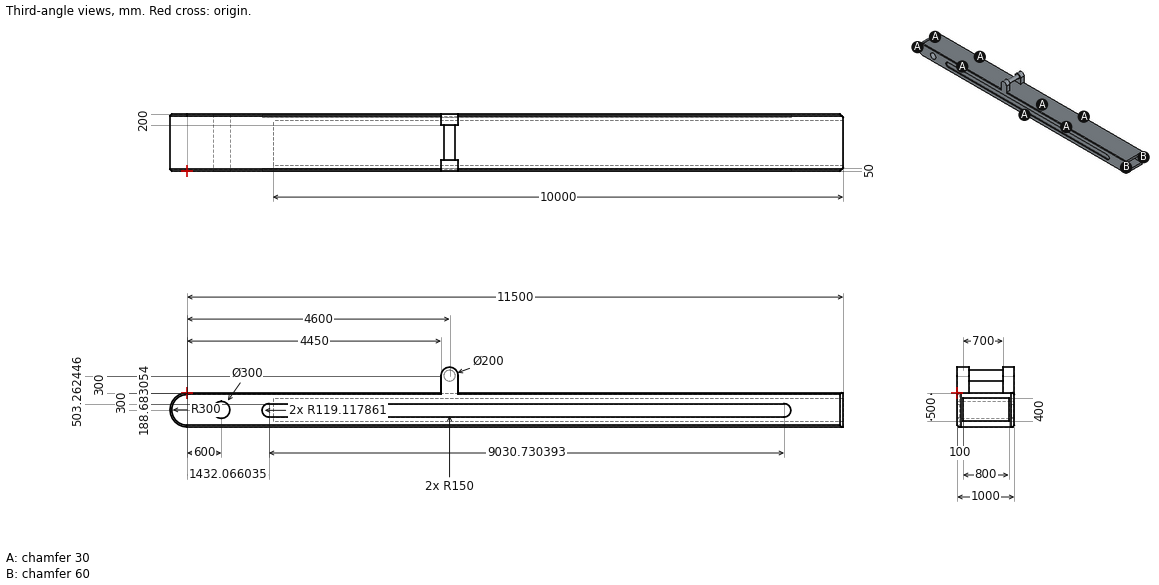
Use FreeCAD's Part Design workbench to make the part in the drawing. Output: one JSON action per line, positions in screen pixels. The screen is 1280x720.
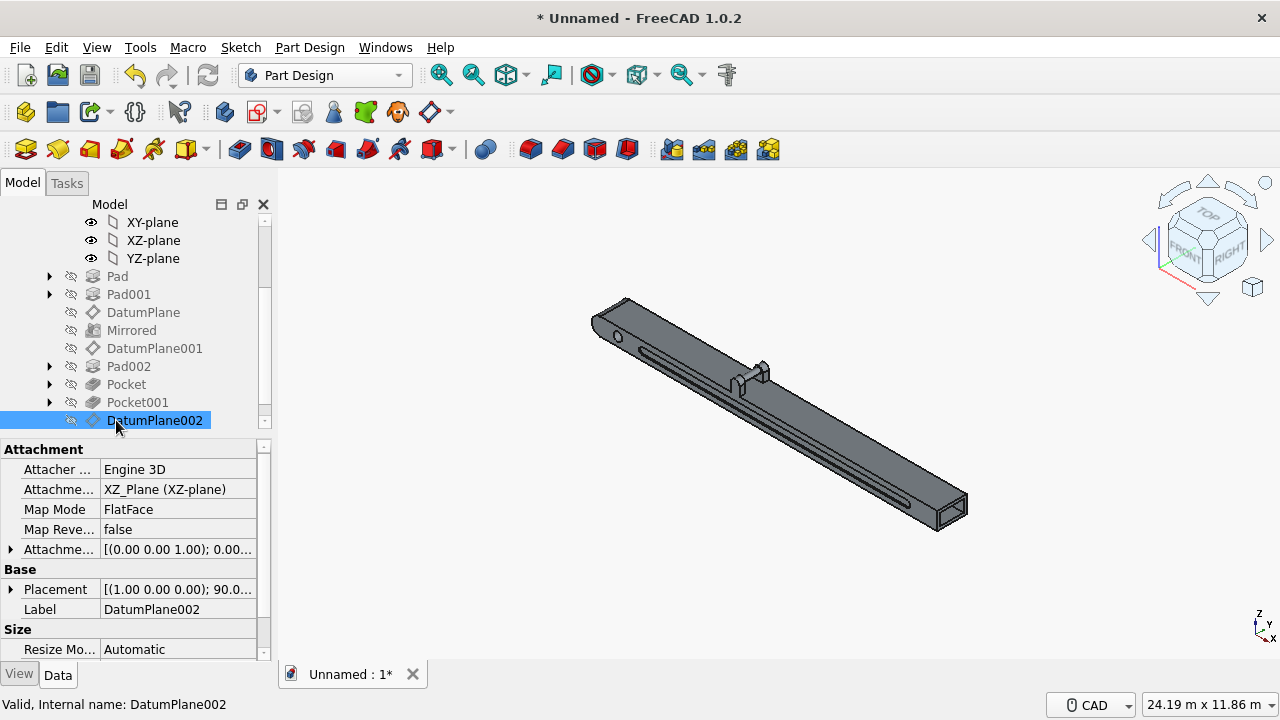
{"action": "left_click", "coordinate": [838, 453]}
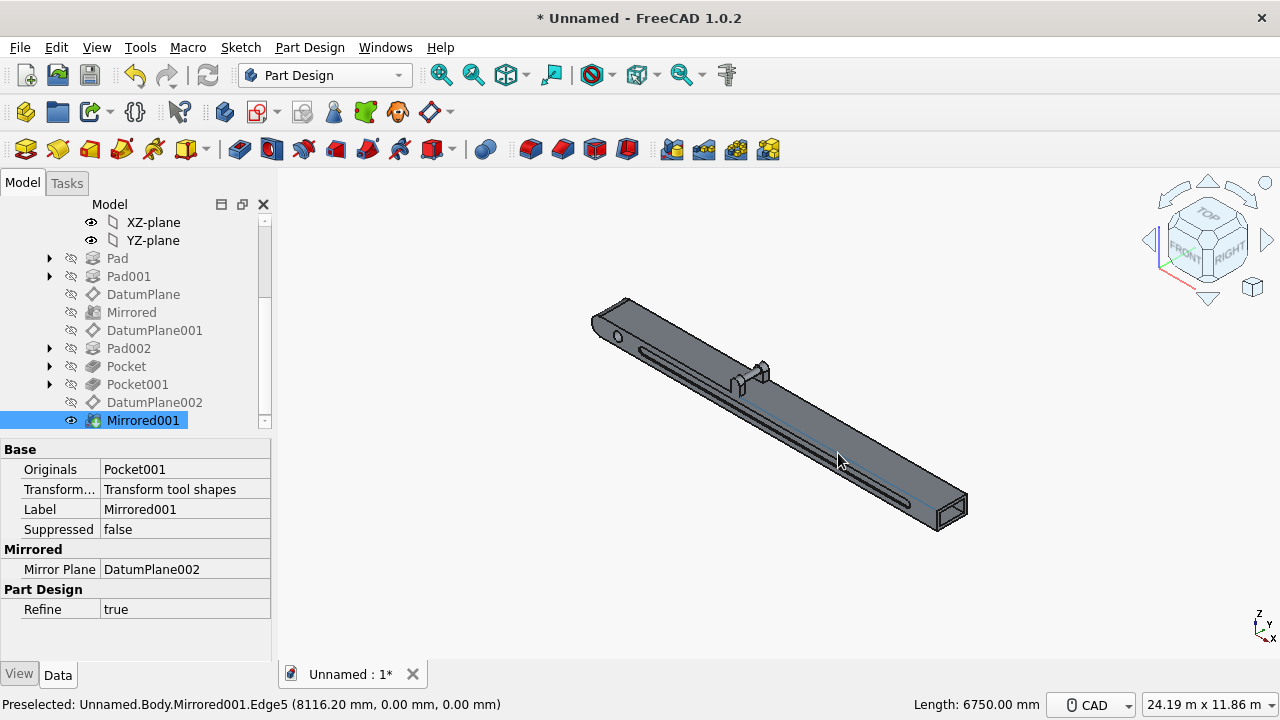
{"action": "left_click", "coordinate": [666, 353], "text": "ctrl"}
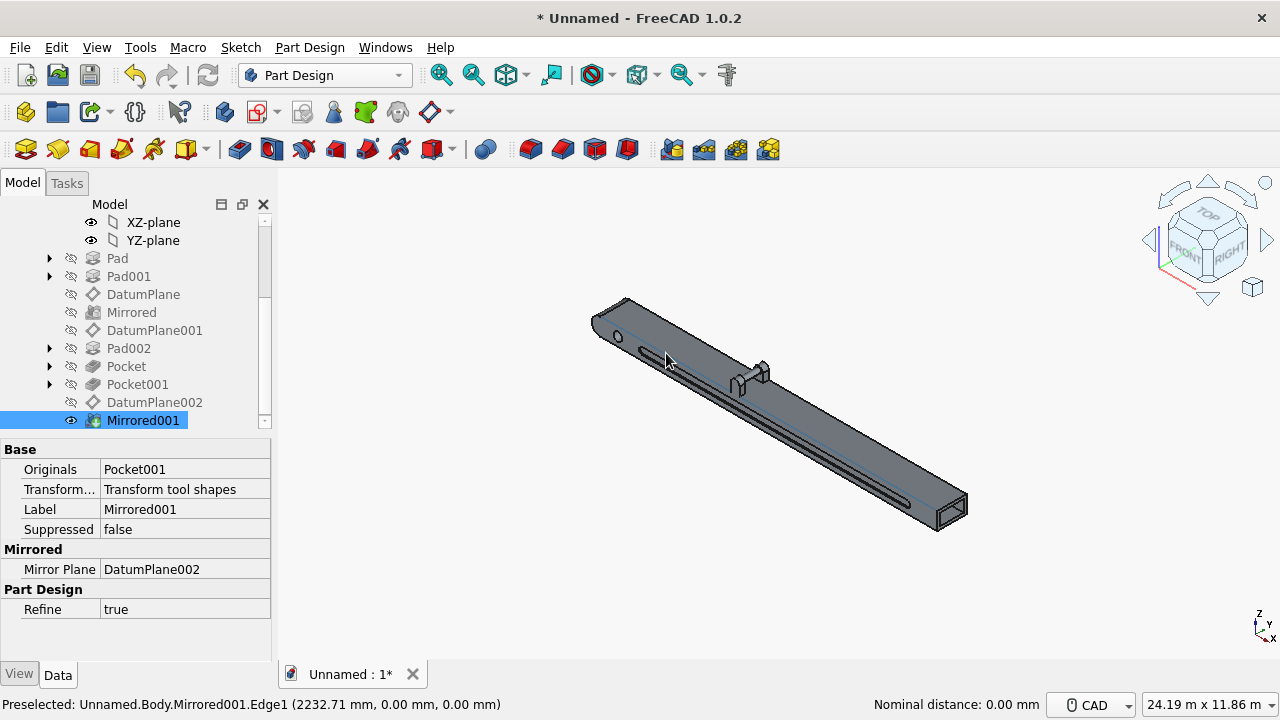
{"action": "left_click", "coordinate": [592, 321], "text": "ctrl"}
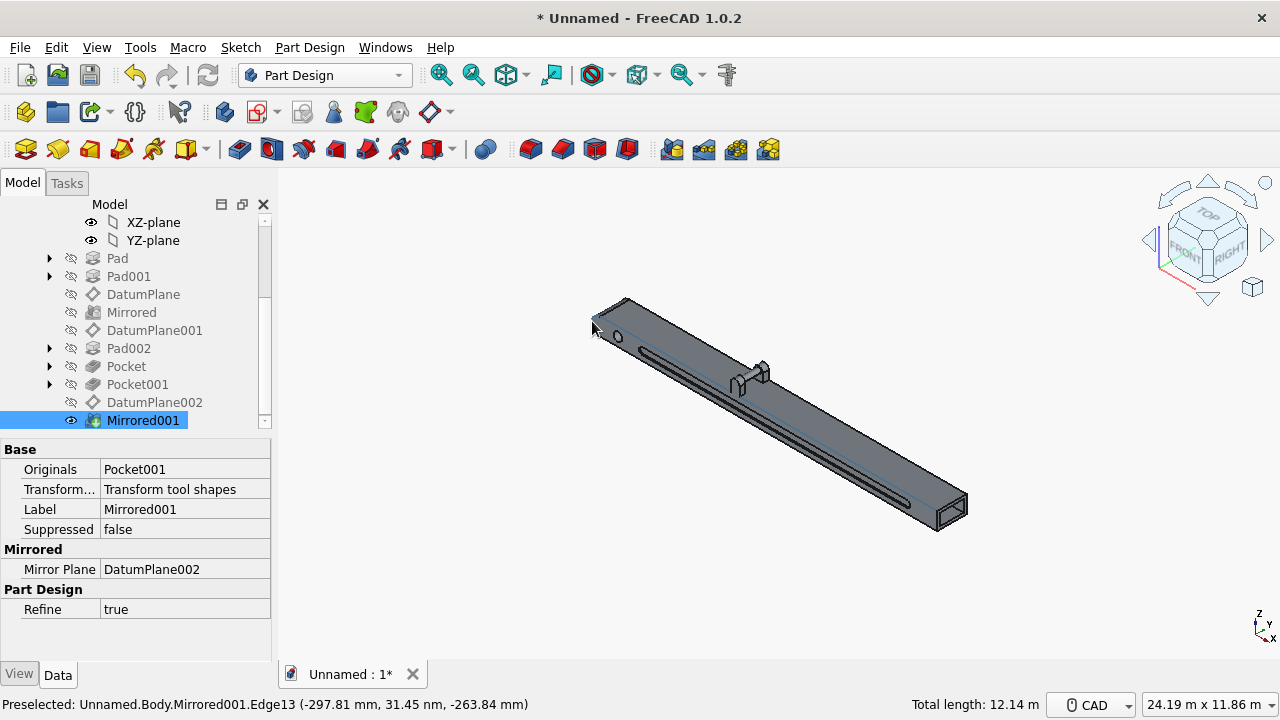
{"action": "key", "text": "2"}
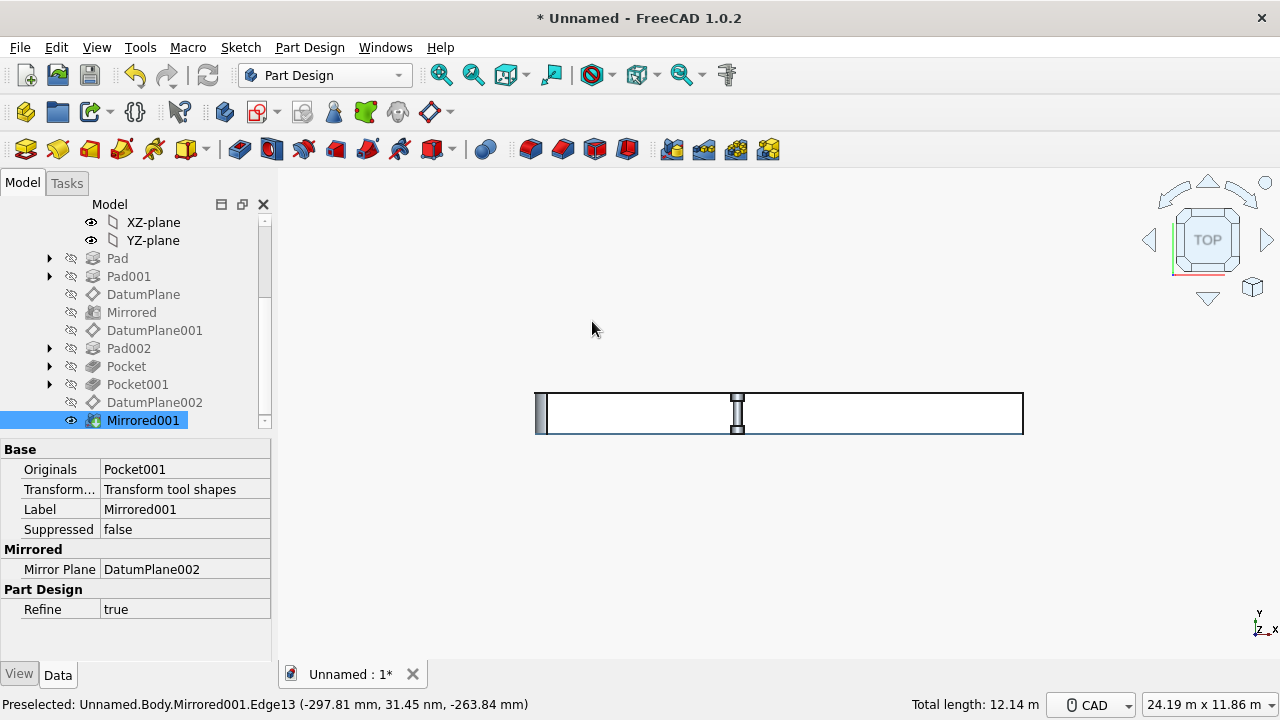
{"action": "left_click", "coordinate": [884, 392], "text": "ctrl"}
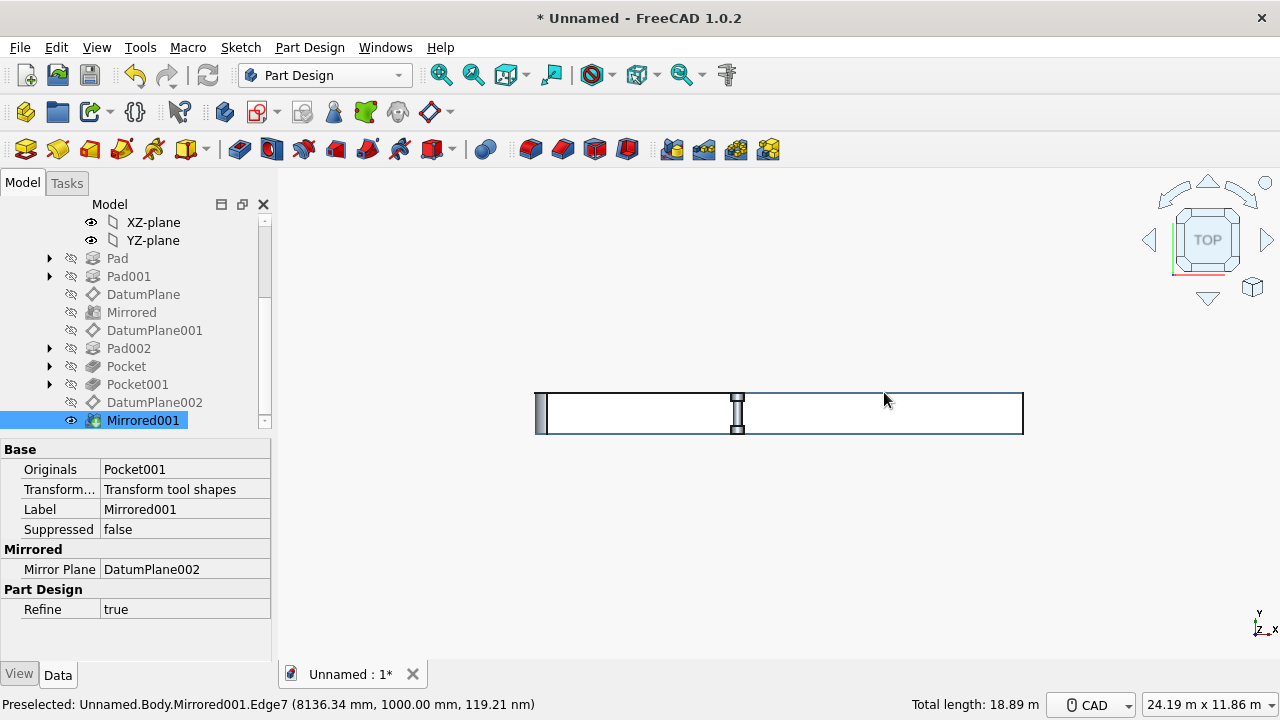
{"action": "left_click", "coordinate": [535, 392], "text": "ctrl"}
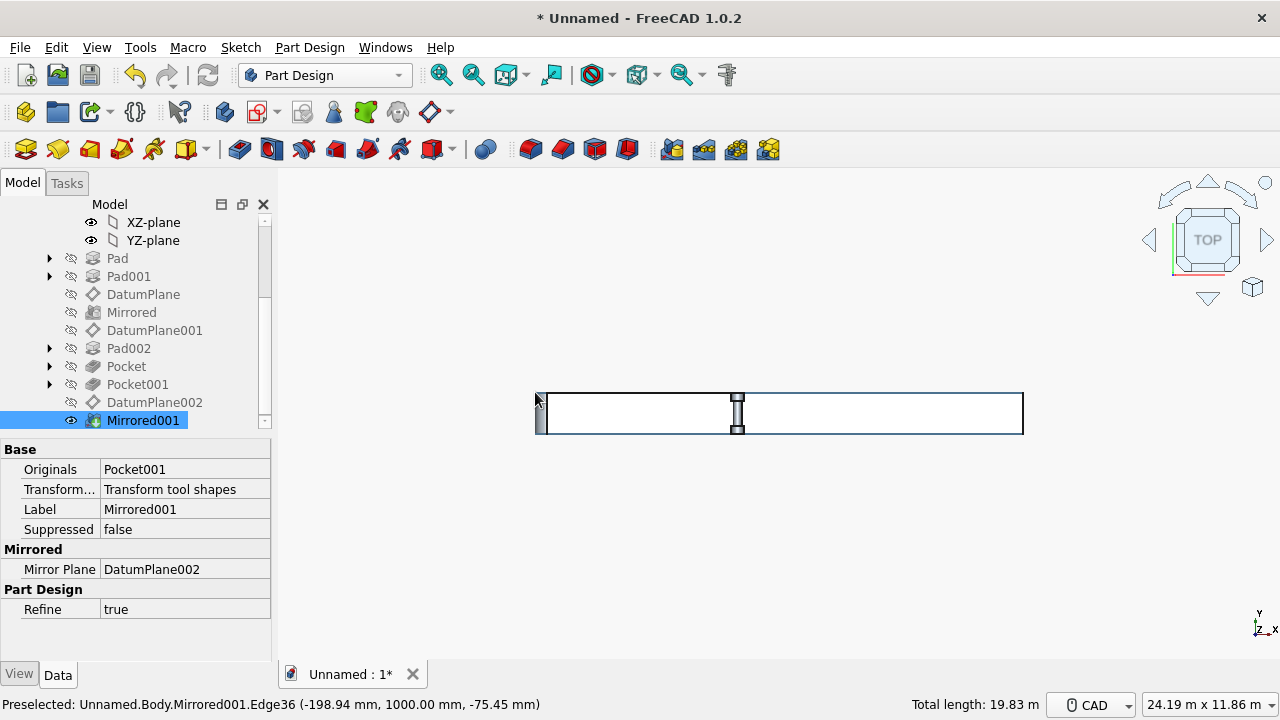
{"action": "left_click", "coordinate": [639, 392], "text": "ctrl"}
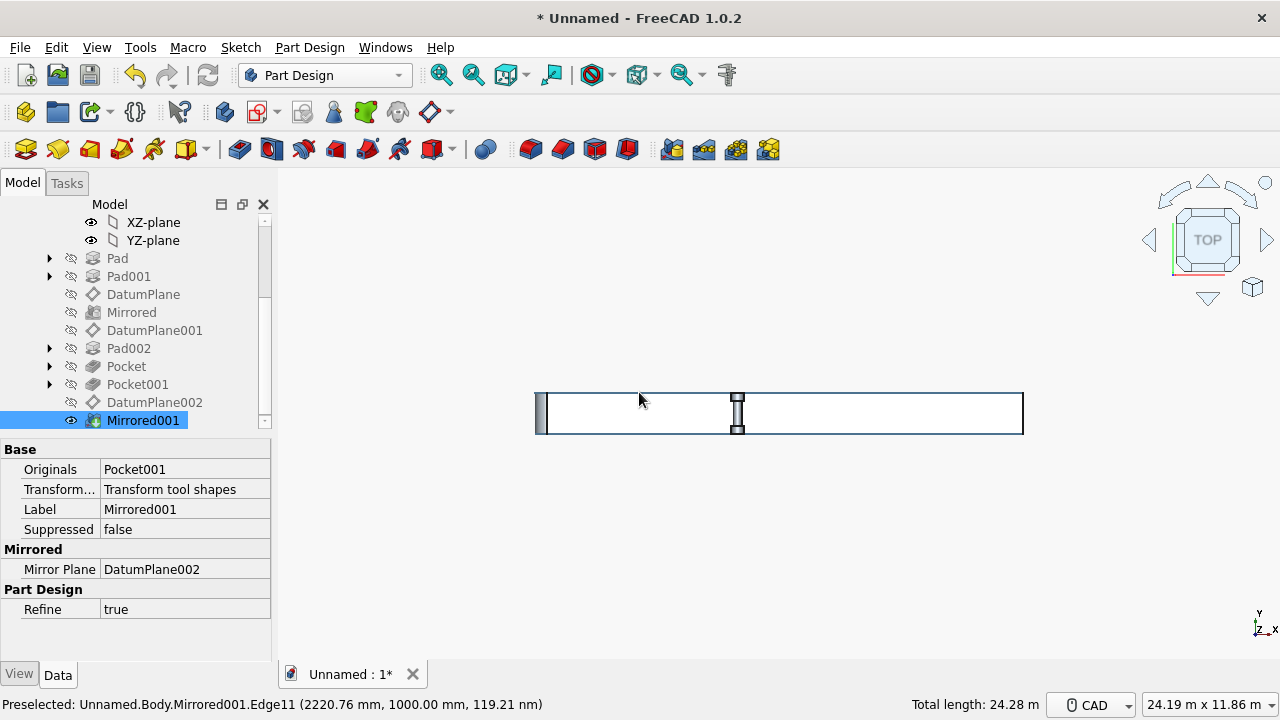
{"action": "key", "text": "0"}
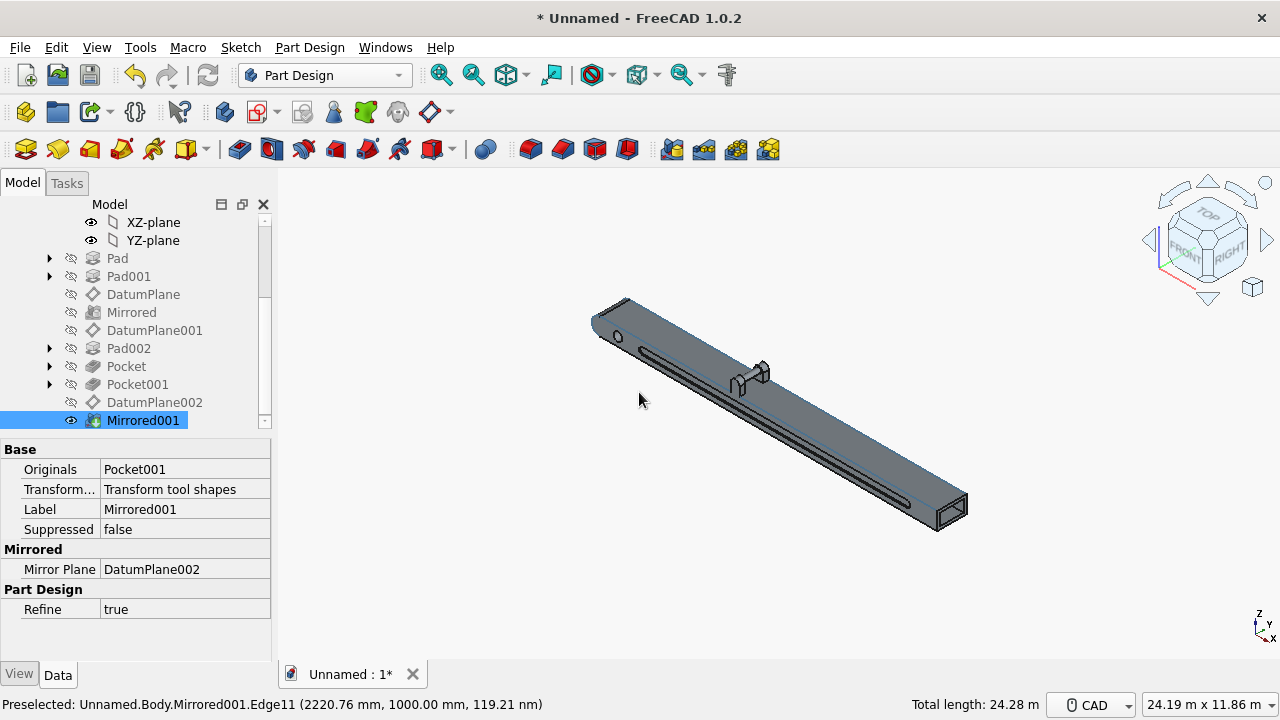
{"action": "key", "text": "1"}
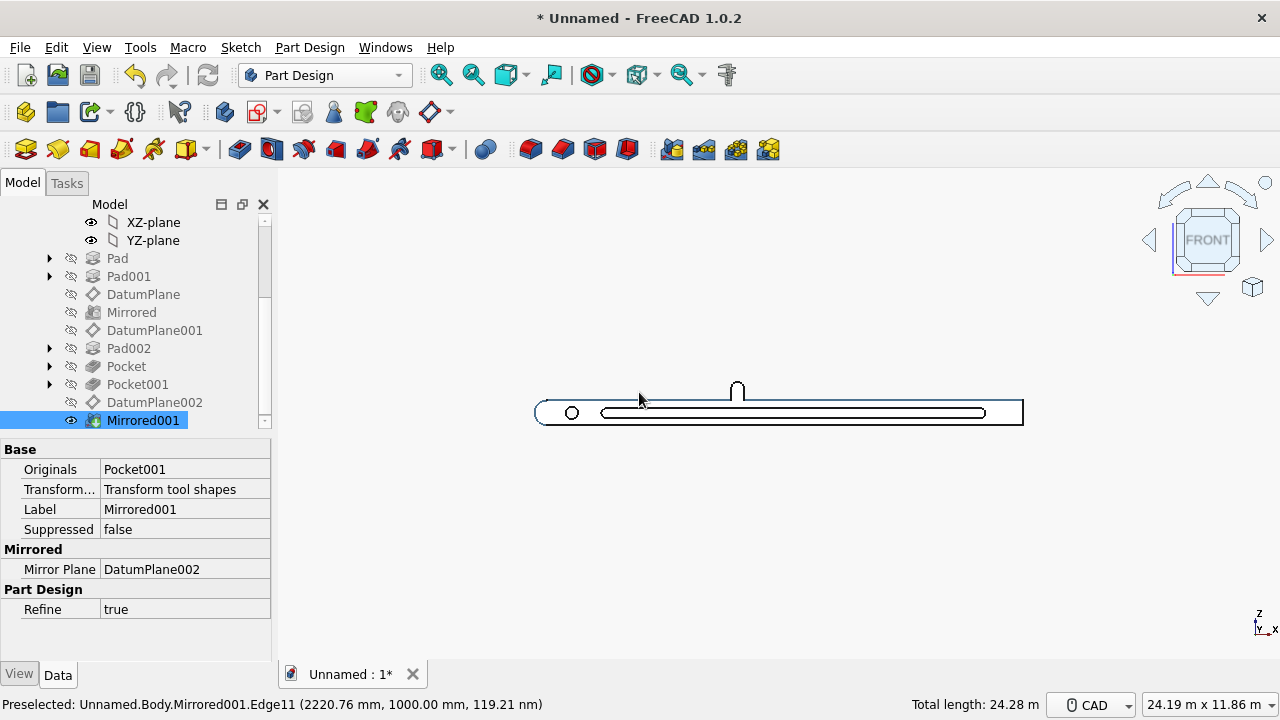
{"action": "key", "text": "3"}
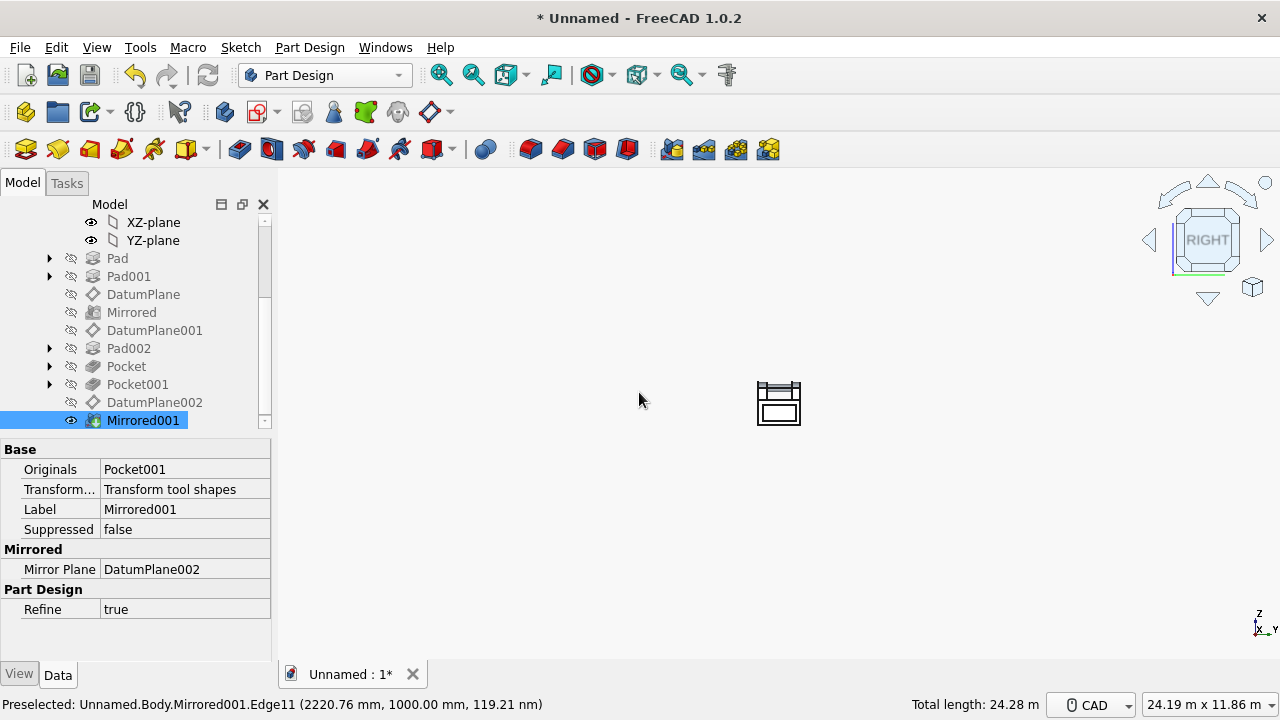
{"action": "left_click", "coordinate": [442, 76]}